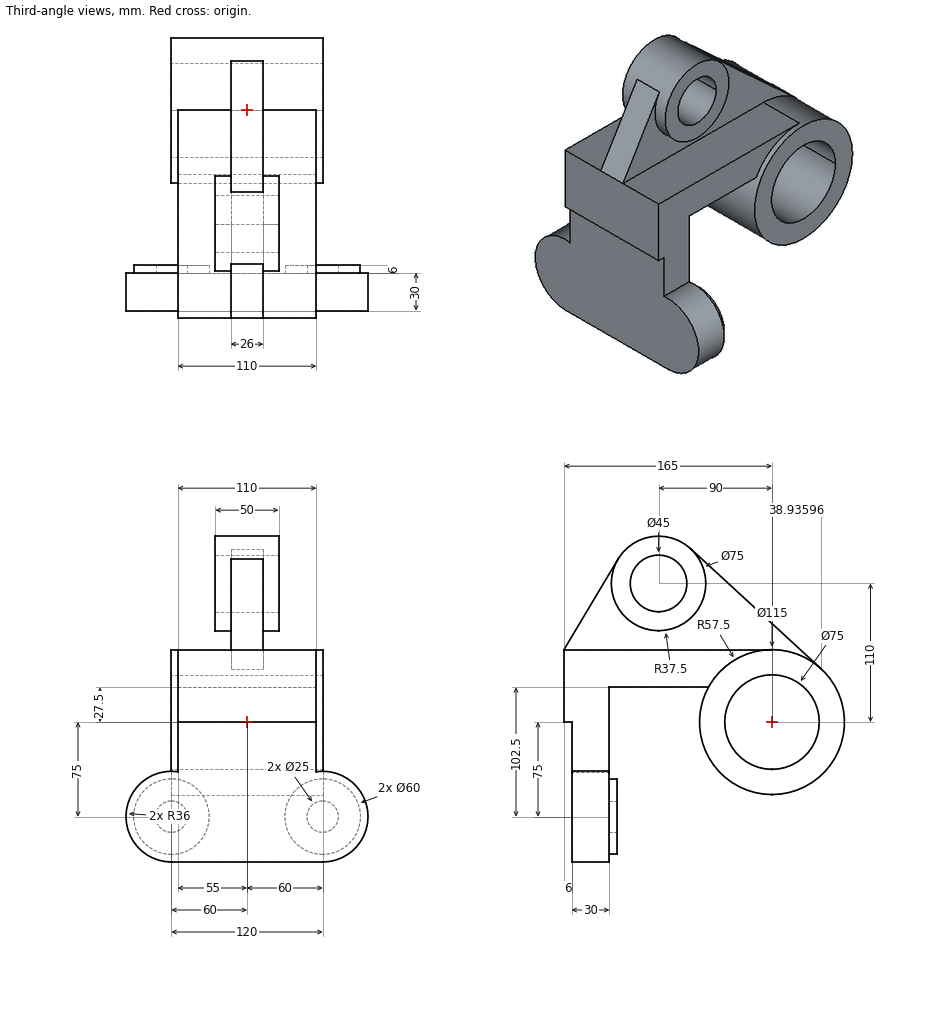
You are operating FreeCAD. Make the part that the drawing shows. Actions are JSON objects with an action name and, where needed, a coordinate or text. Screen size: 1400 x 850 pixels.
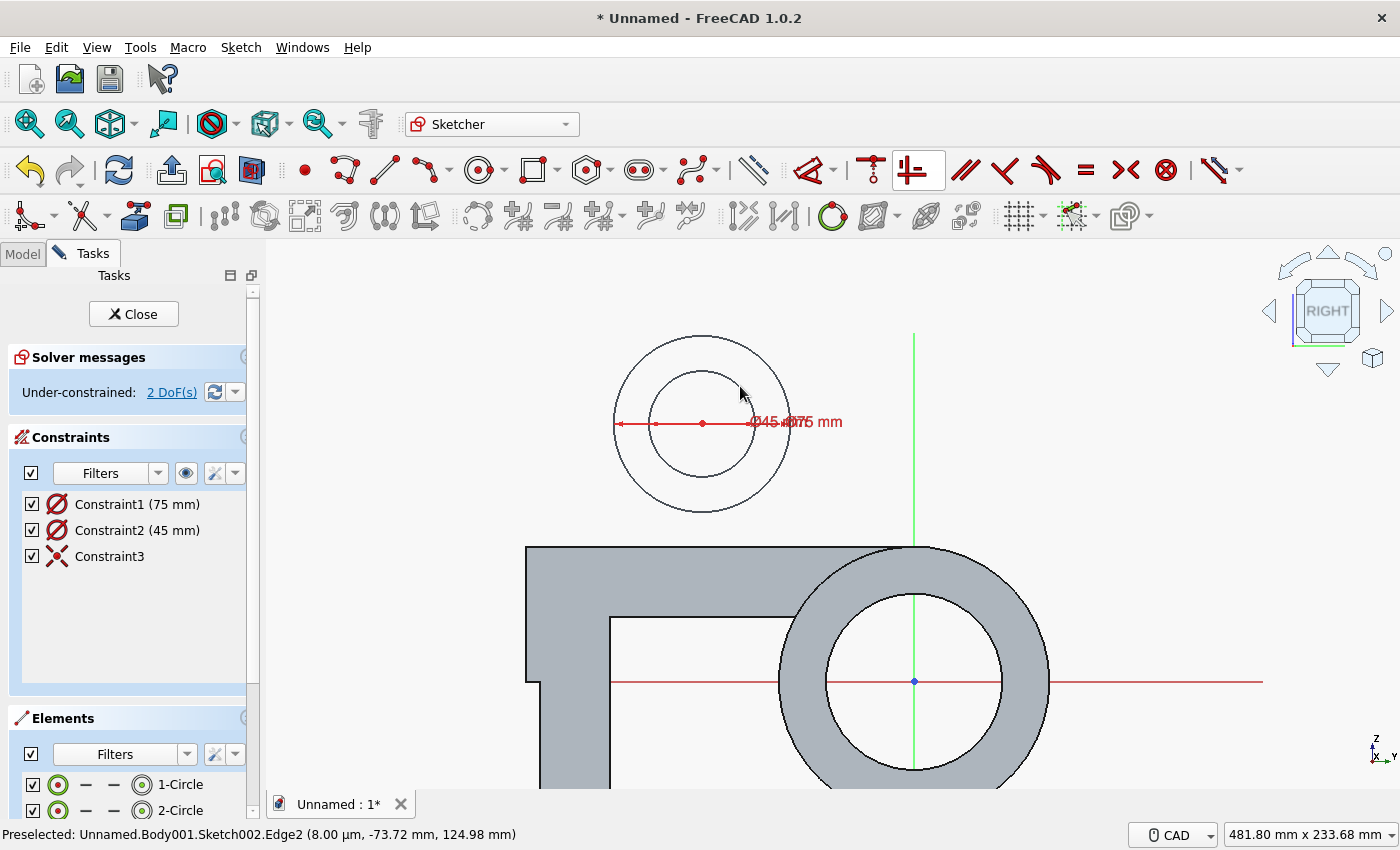
{"action": "key", "text": "d"}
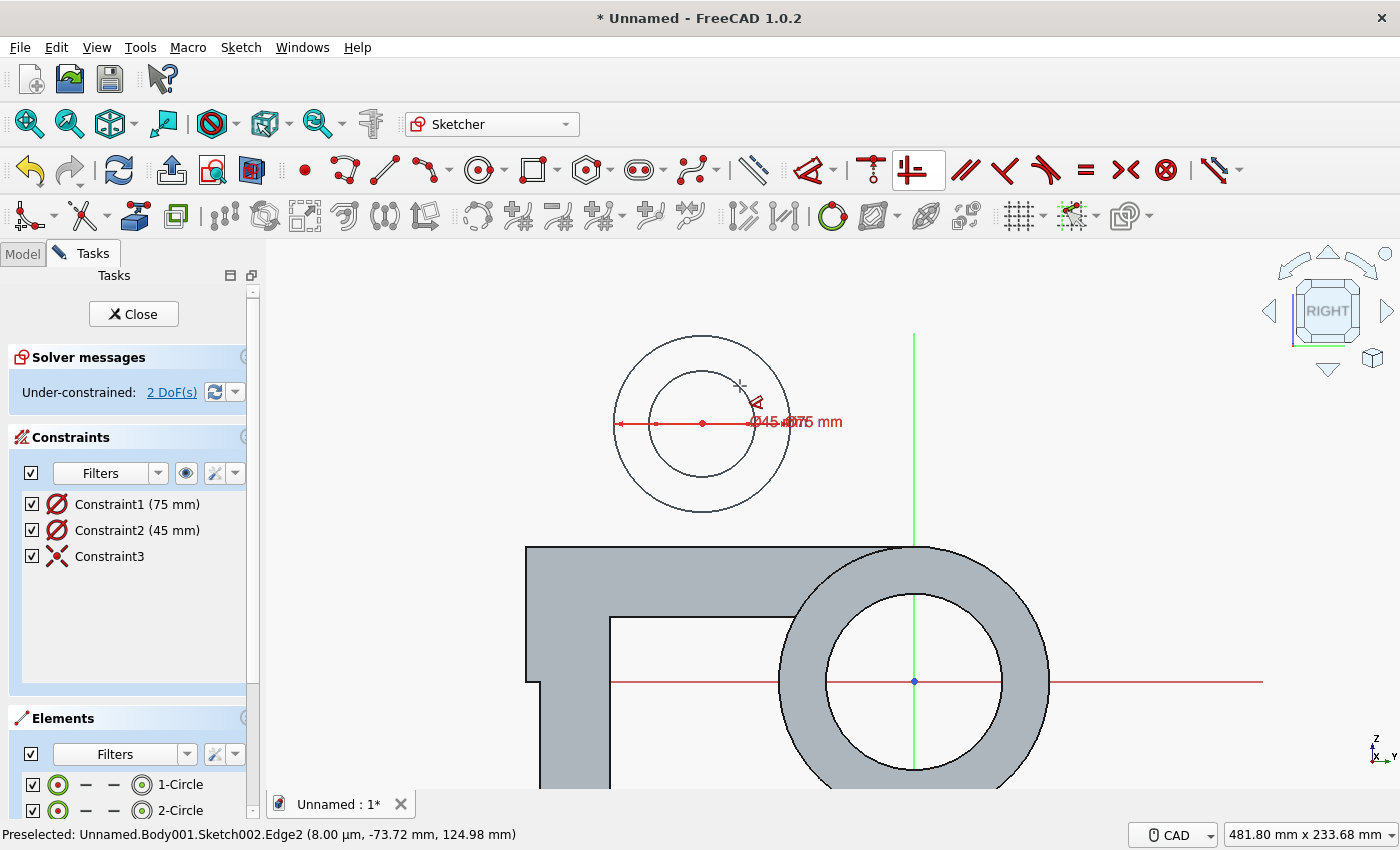
{"action": "left_click", "coordinate": [702, 424]}
{"action": "left_click", "coordinate": [808, 716]}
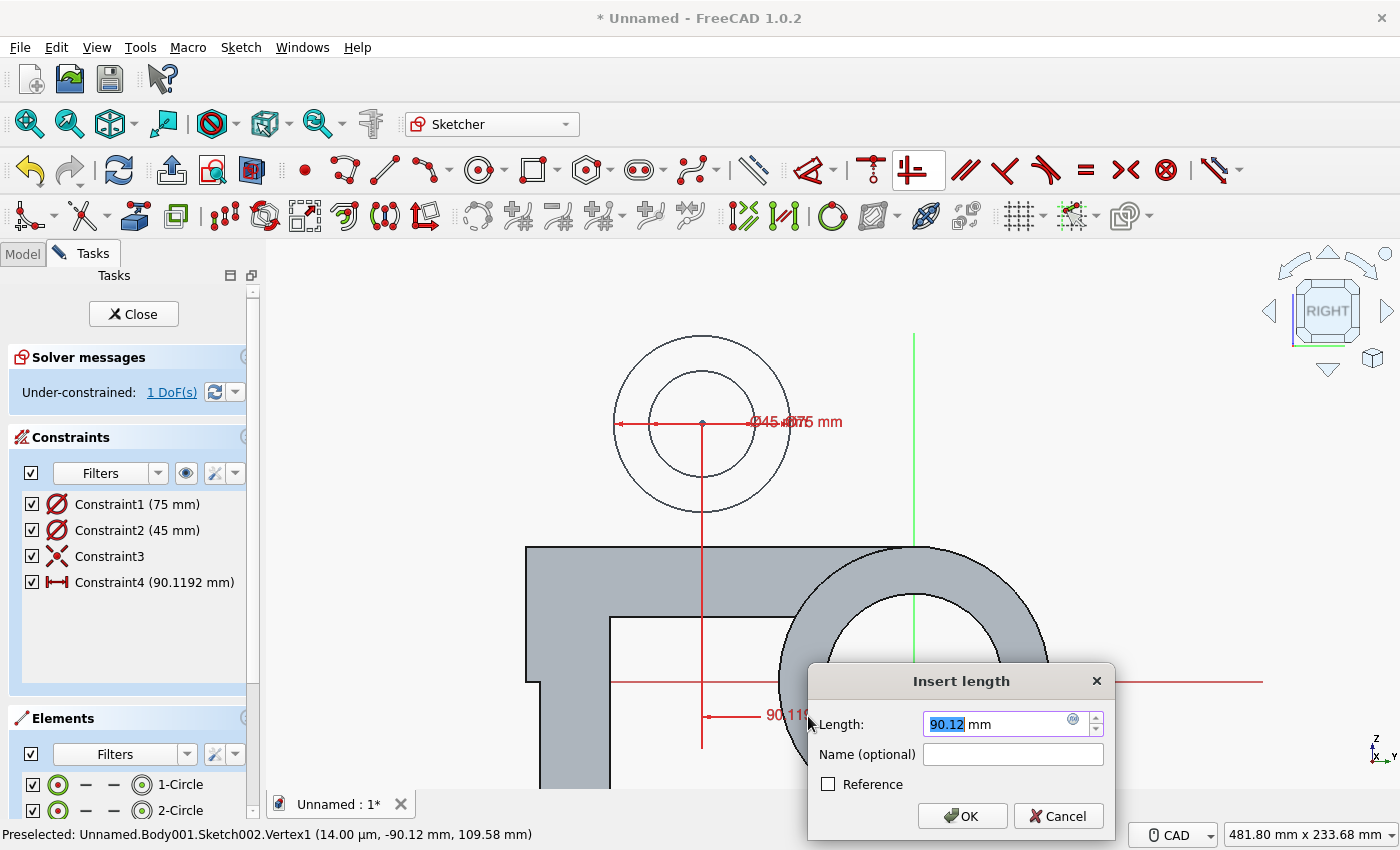
{"action": "type", "text": "90"}
{"action": "key", "text": "Return"}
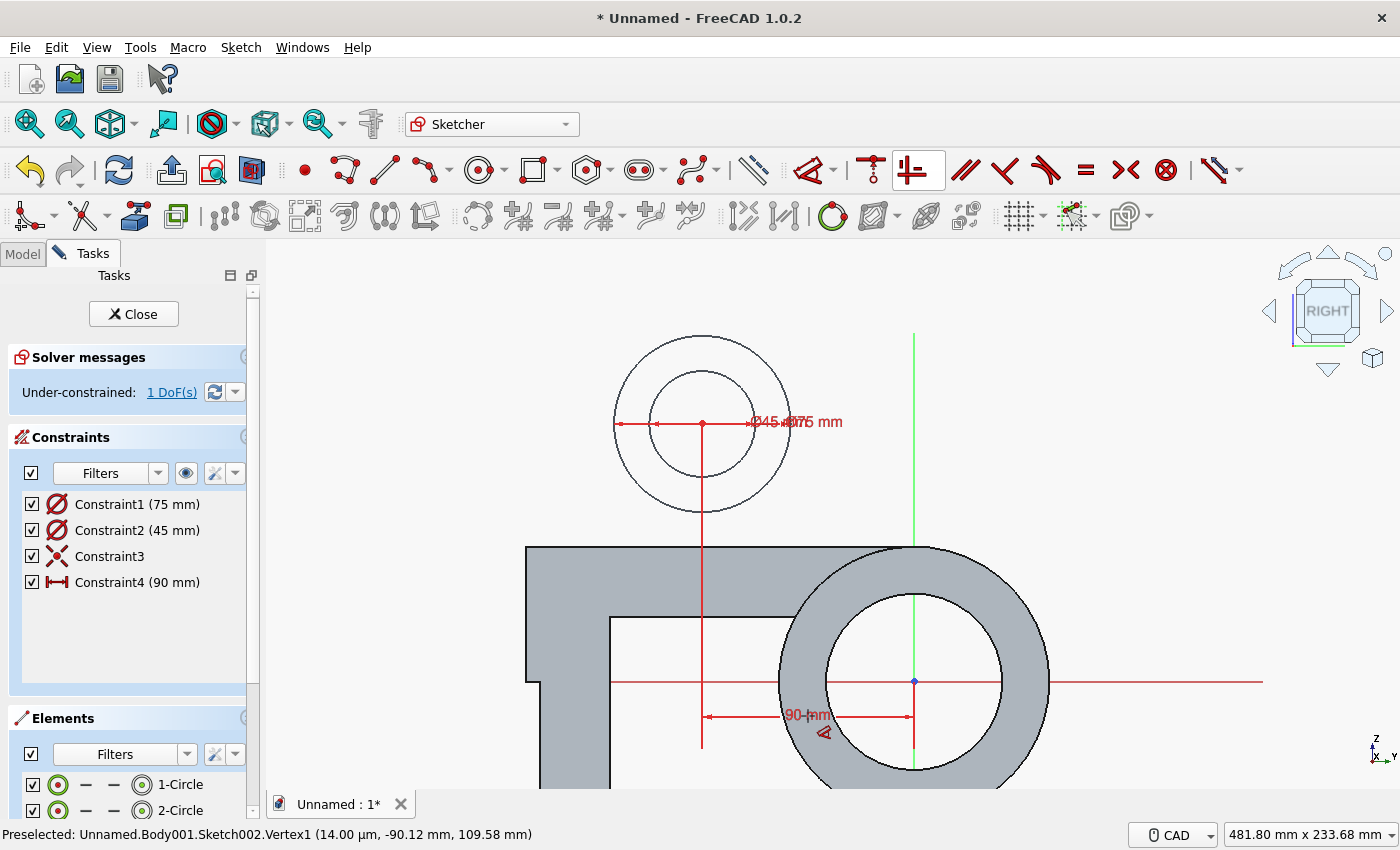
{"action": "left_click", "coordinate": [702, 424]}
{"action": "left_click", "coordinate": [948, 553]}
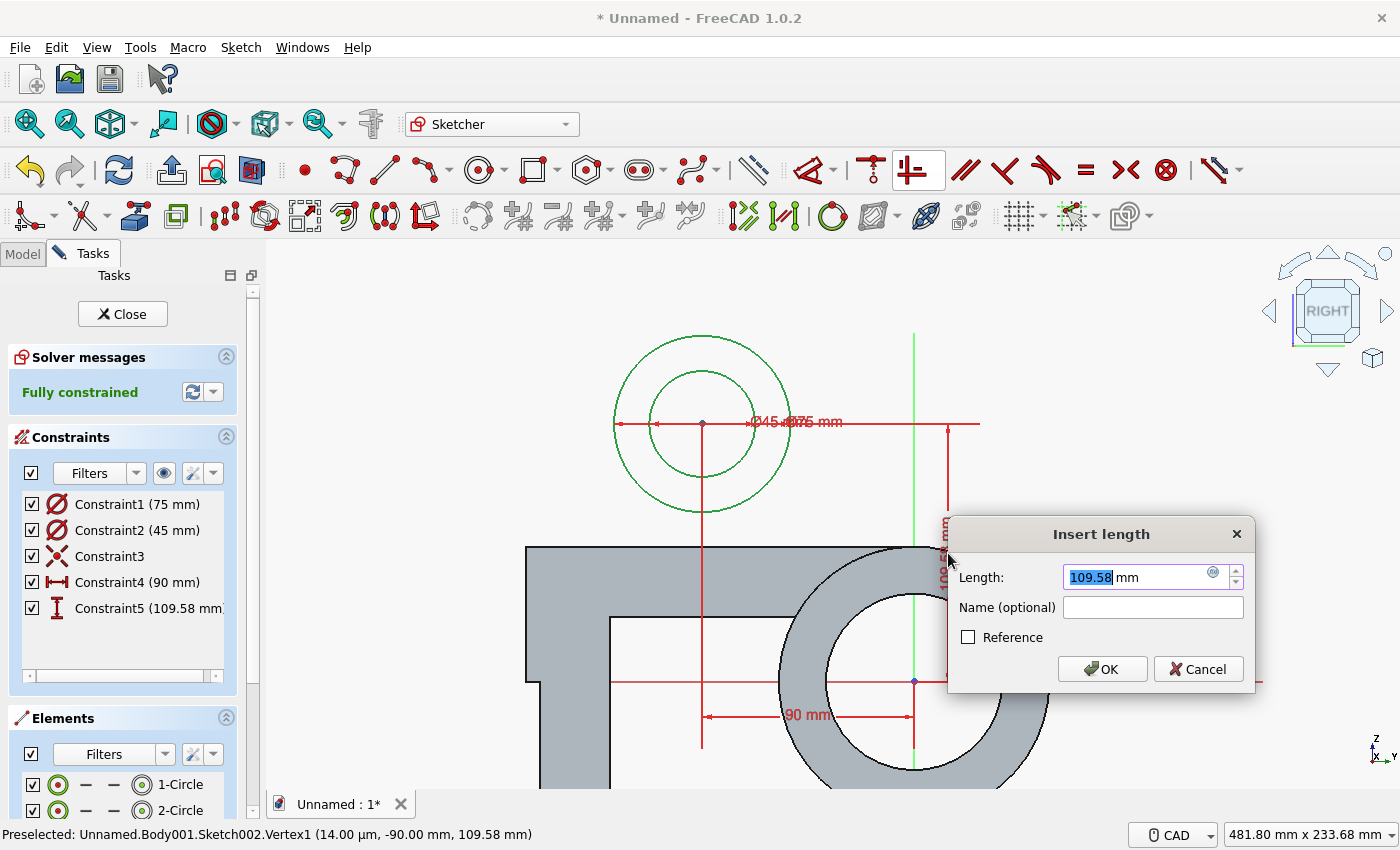
{"action": "type", "text": "110"}
{"action": "key", "text": "Return"}
{"action": "key", "text": "Escape"}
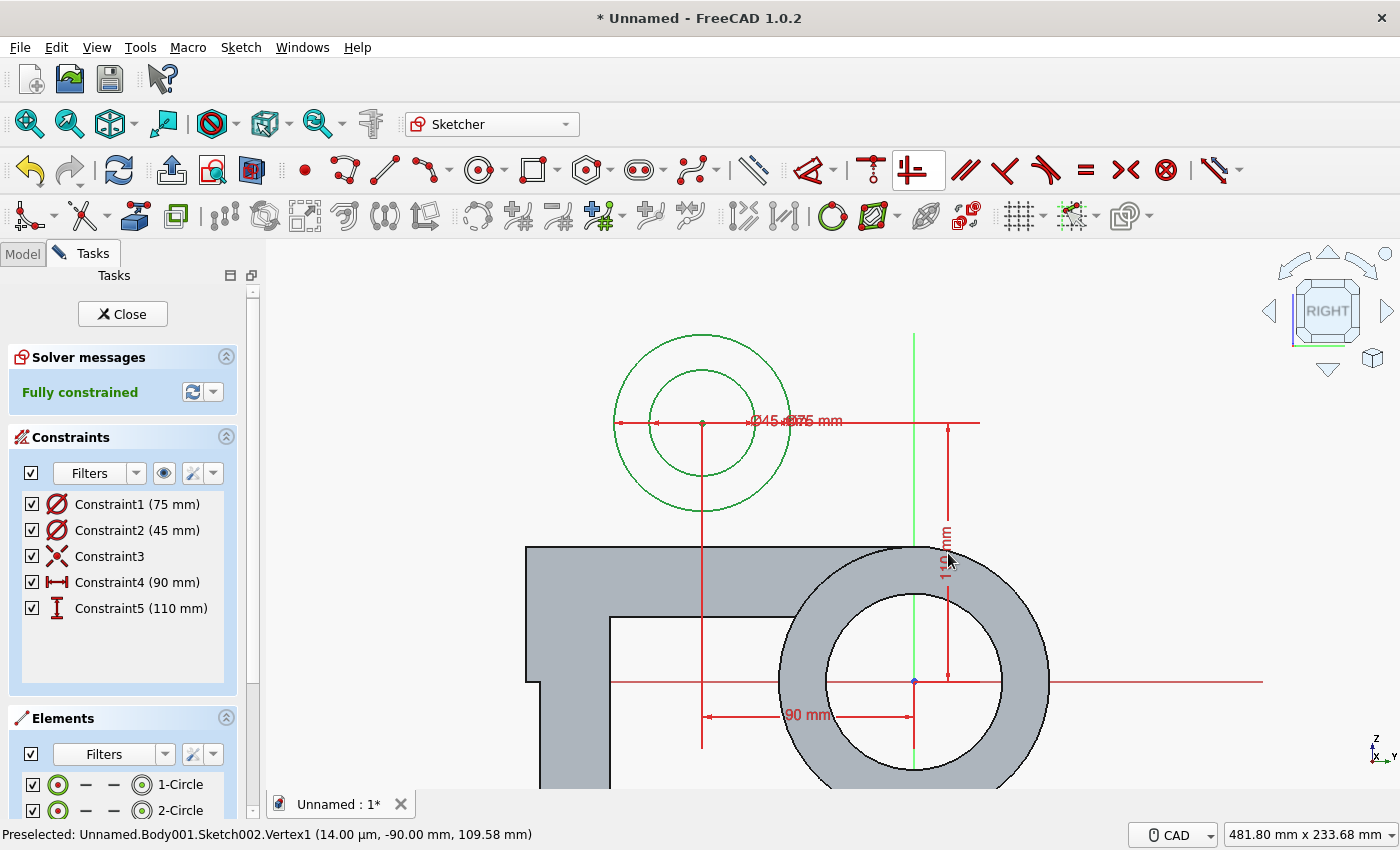
{"action": "left_click", "coordinate": [123, 314]}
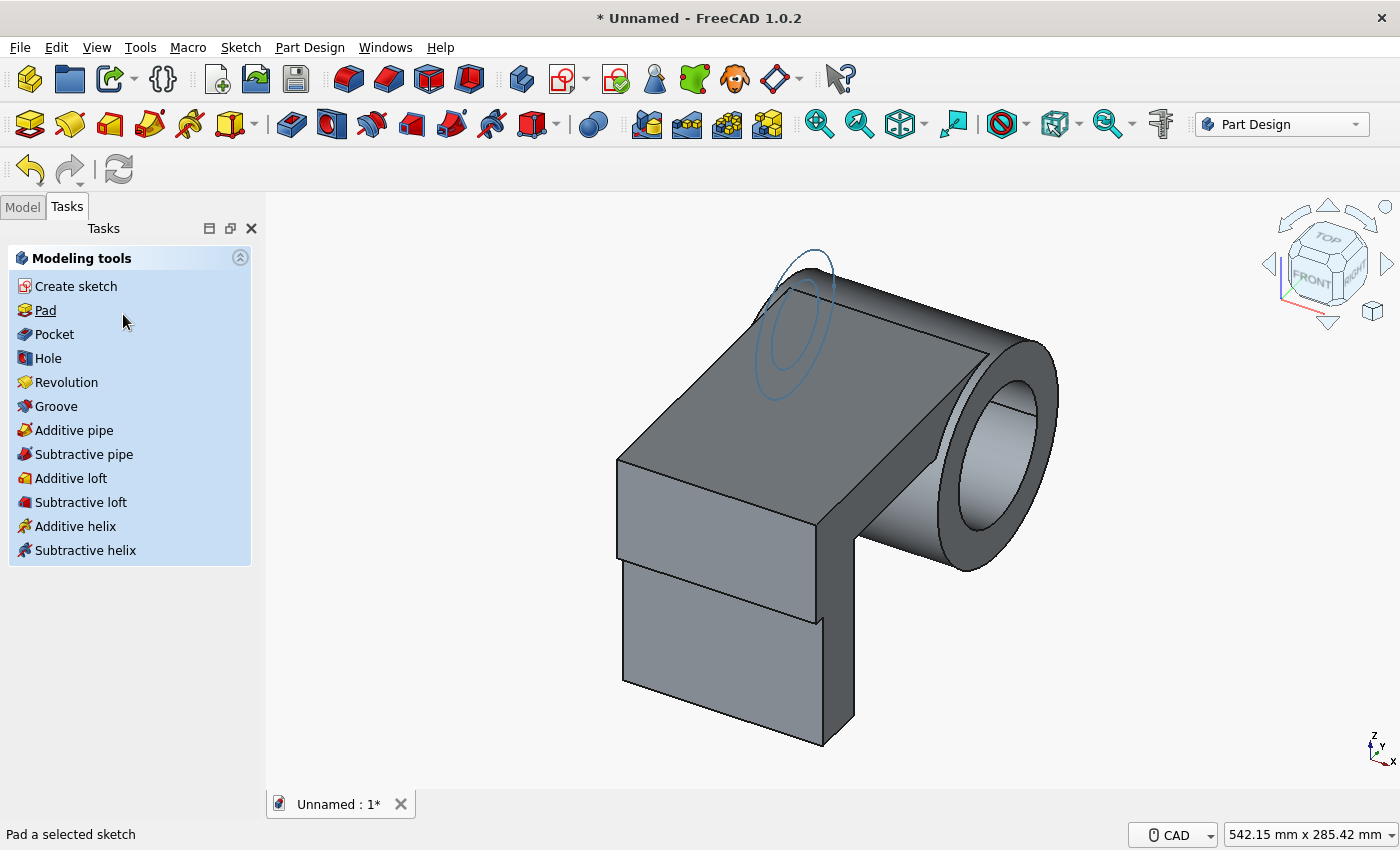
{"action": "left_click", "coordinate": [30, 124]}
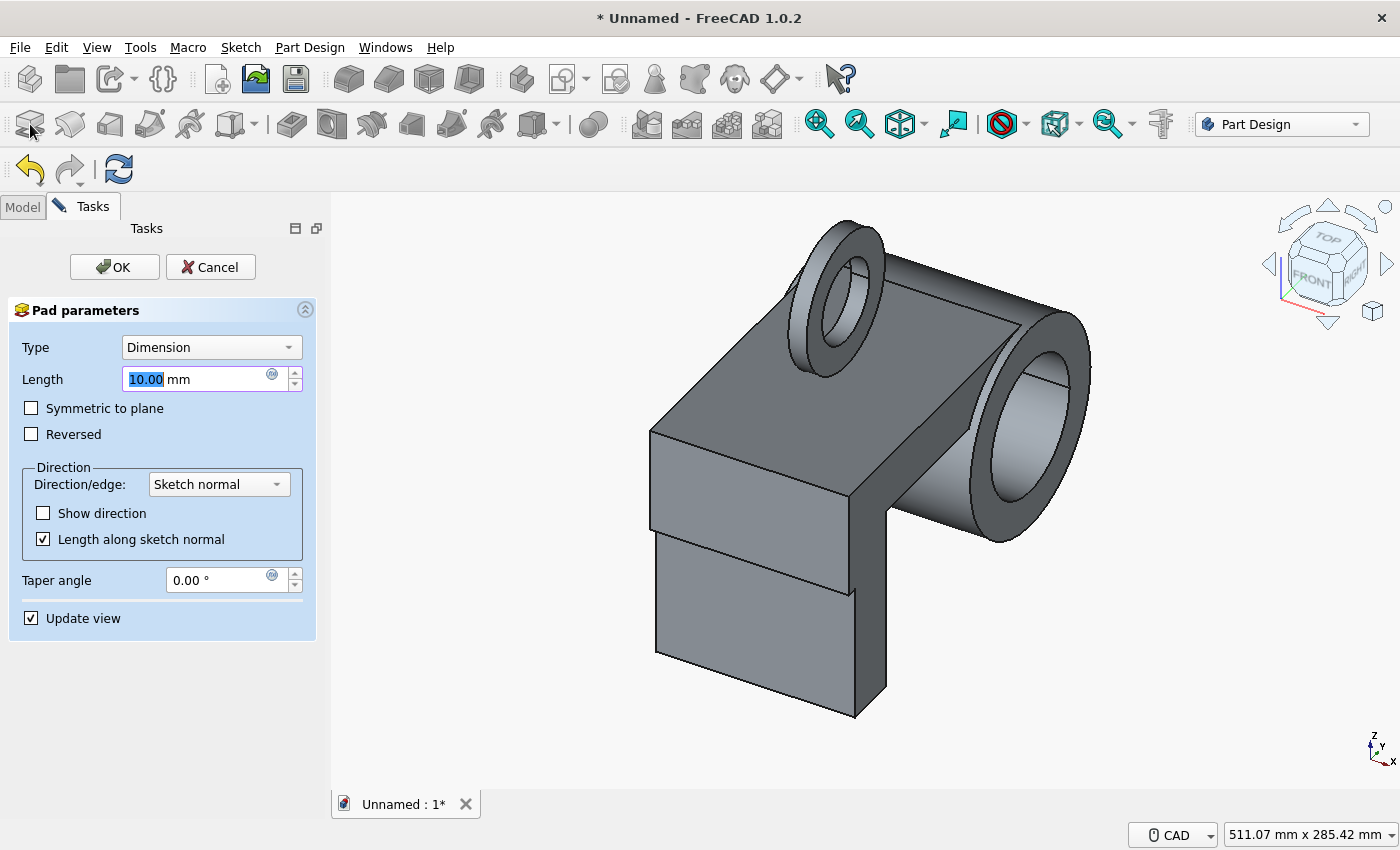
{"action": "type", "text": "50"}
{"action": "key", "text": "Tab"}